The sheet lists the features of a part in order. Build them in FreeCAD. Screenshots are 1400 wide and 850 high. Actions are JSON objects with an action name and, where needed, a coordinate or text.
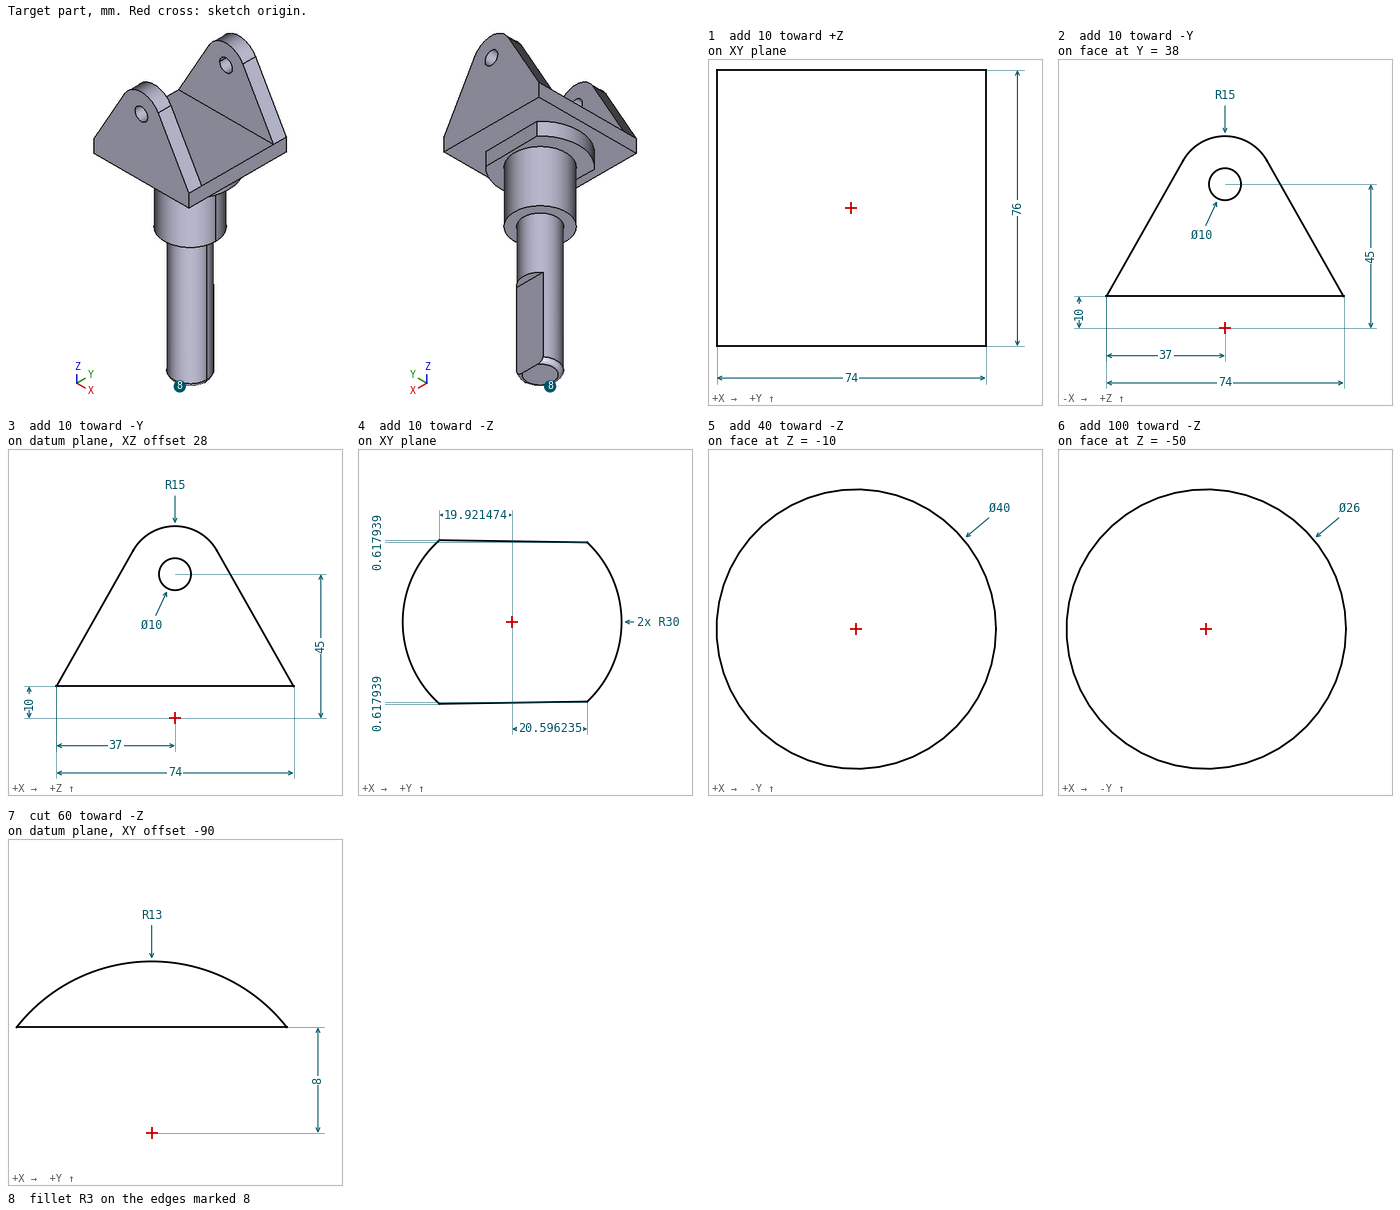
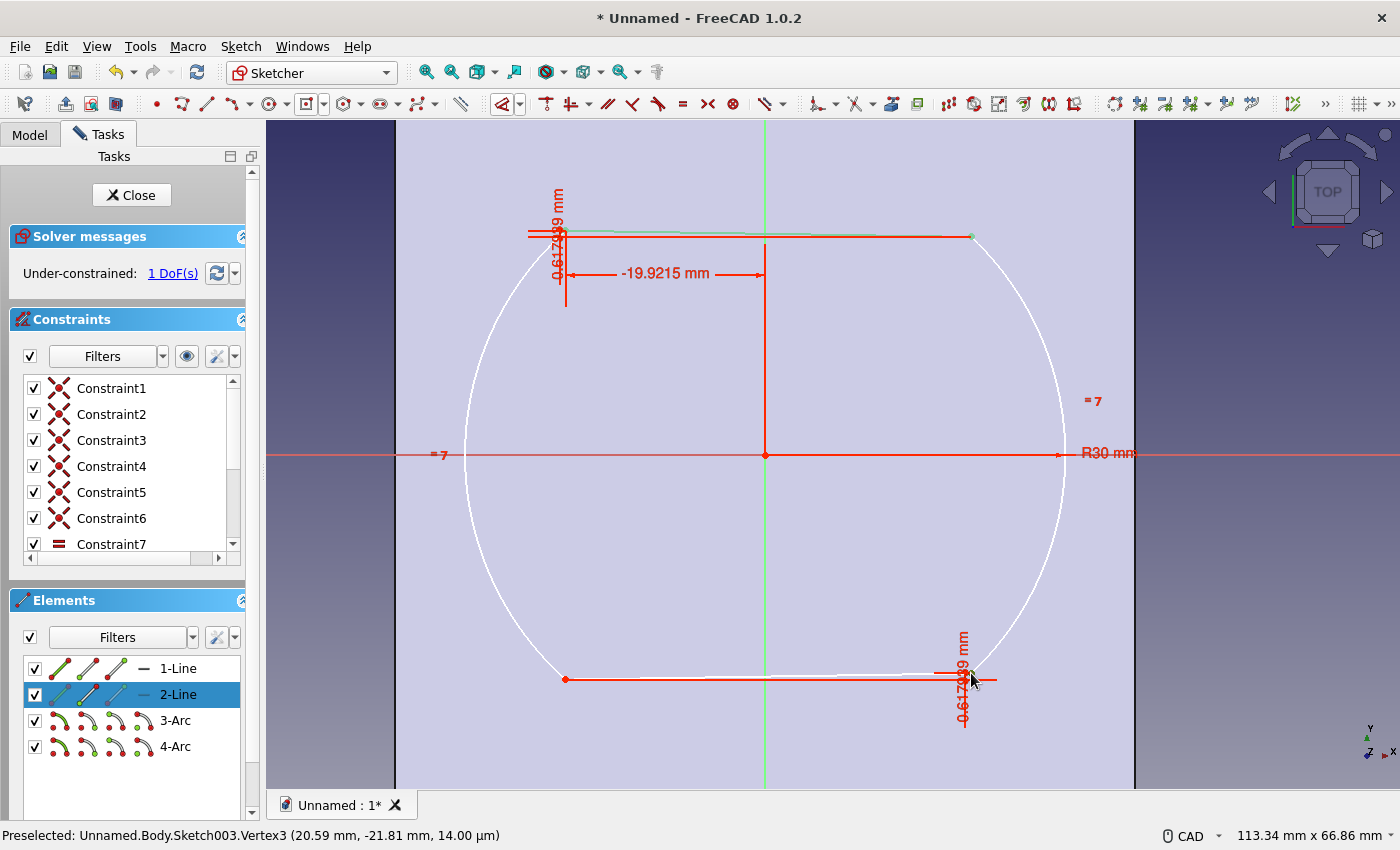
{"action": "left_click", "coordinate": [520, 104]}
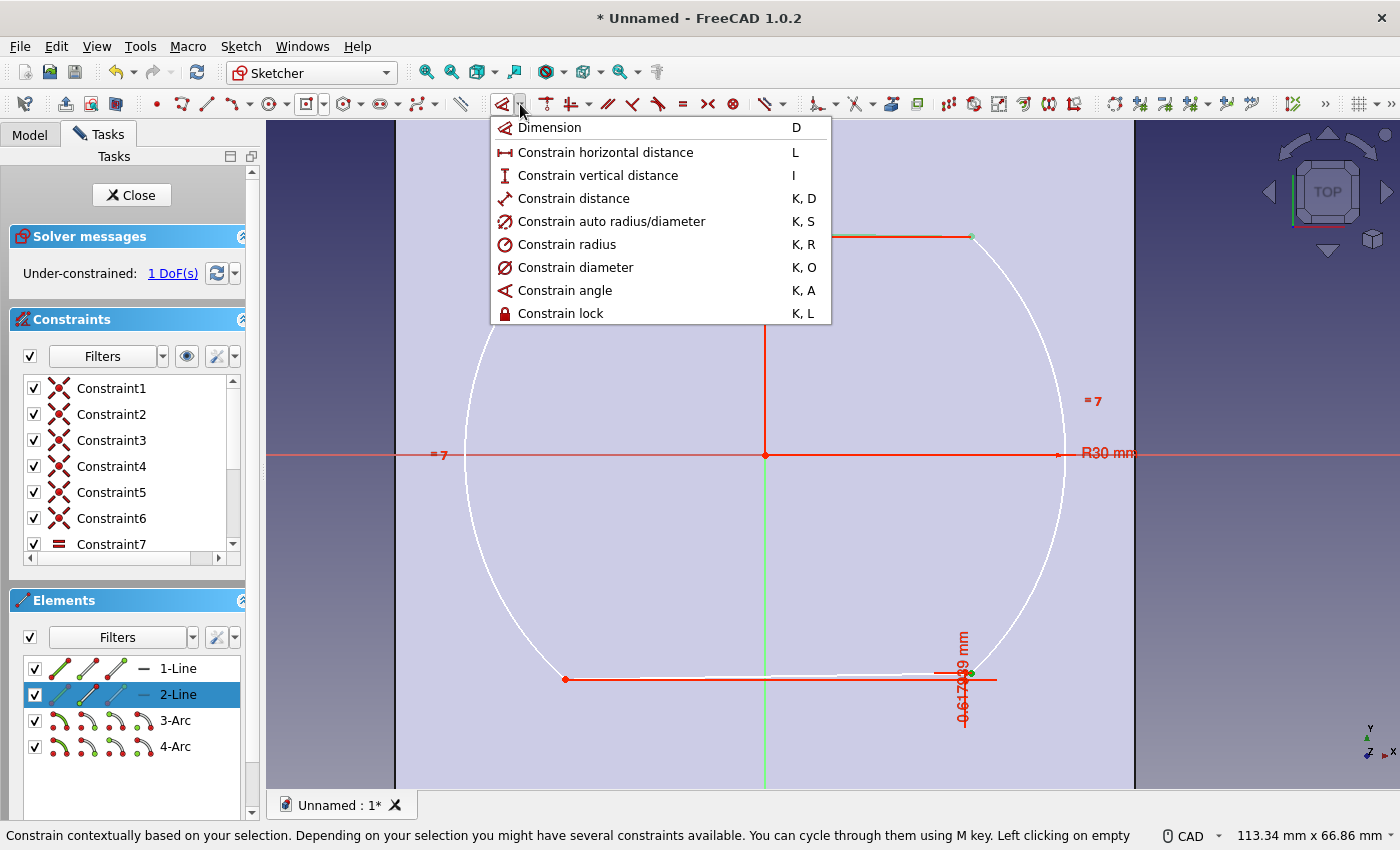
{"action": "left_click", "coordinate": [661, 152]}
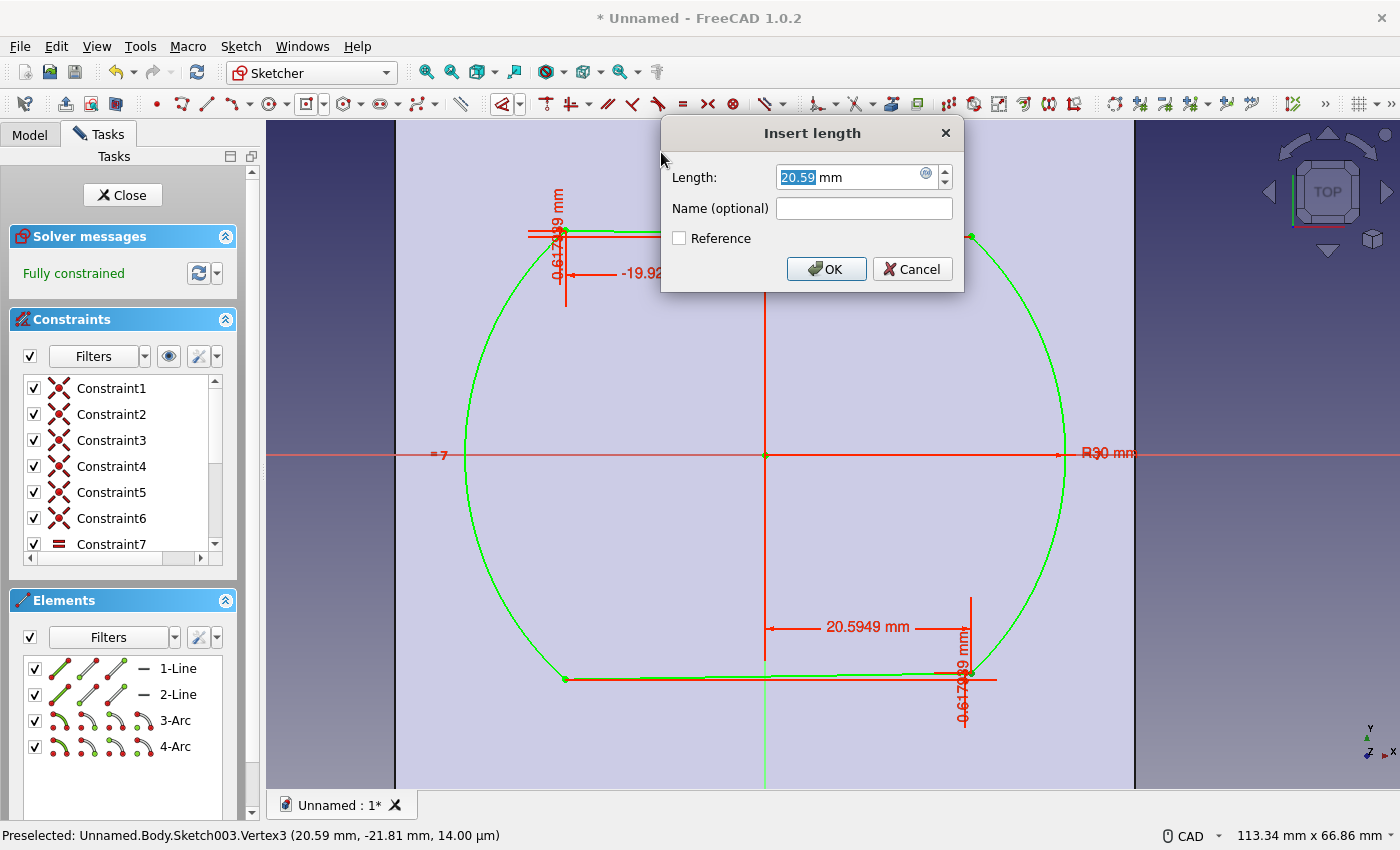
{"action": "type", "text": "20.596235"}
{"action": "key", "text": "Return"}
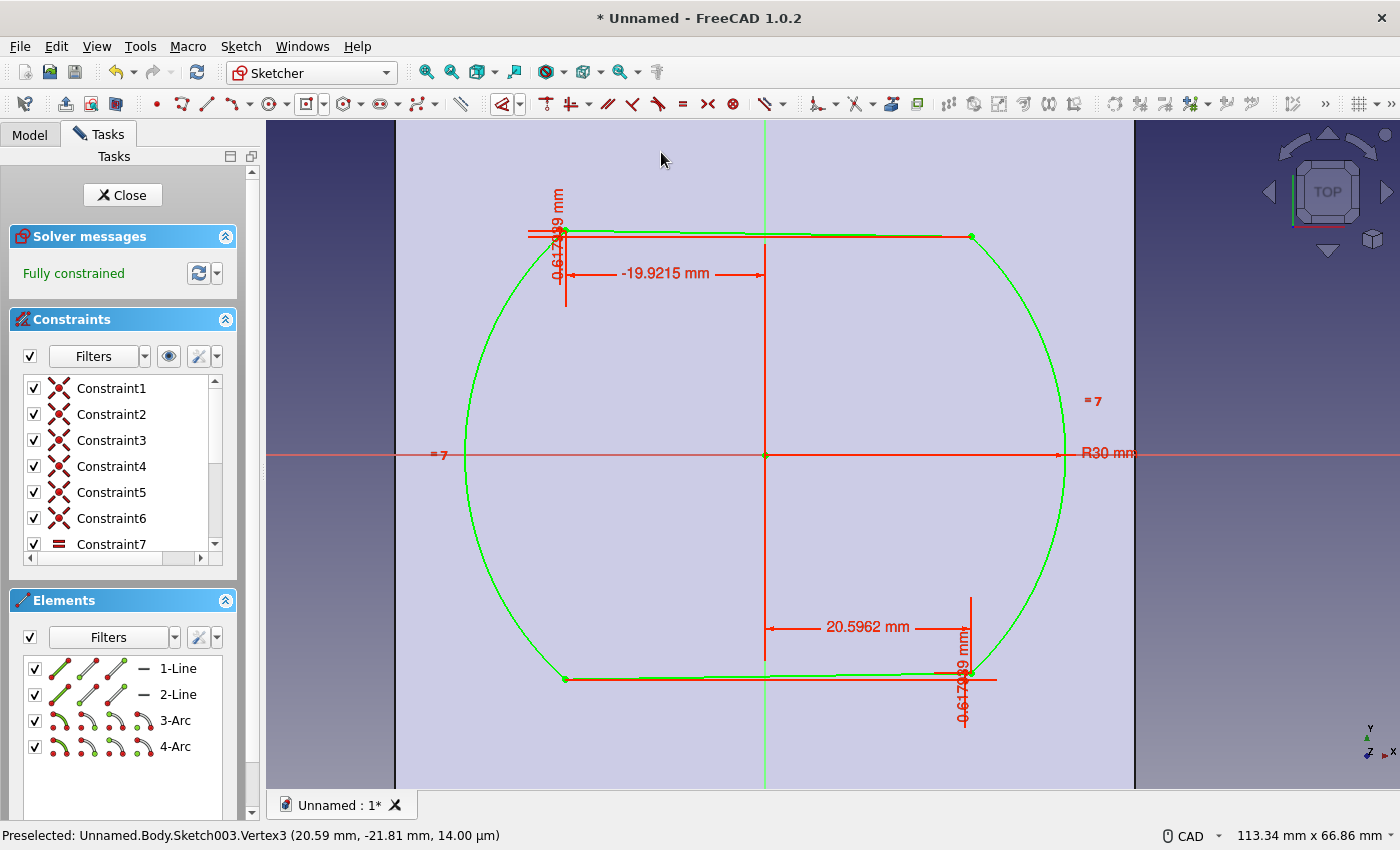
{"action": "left_click", "coordinate": [123, 195]}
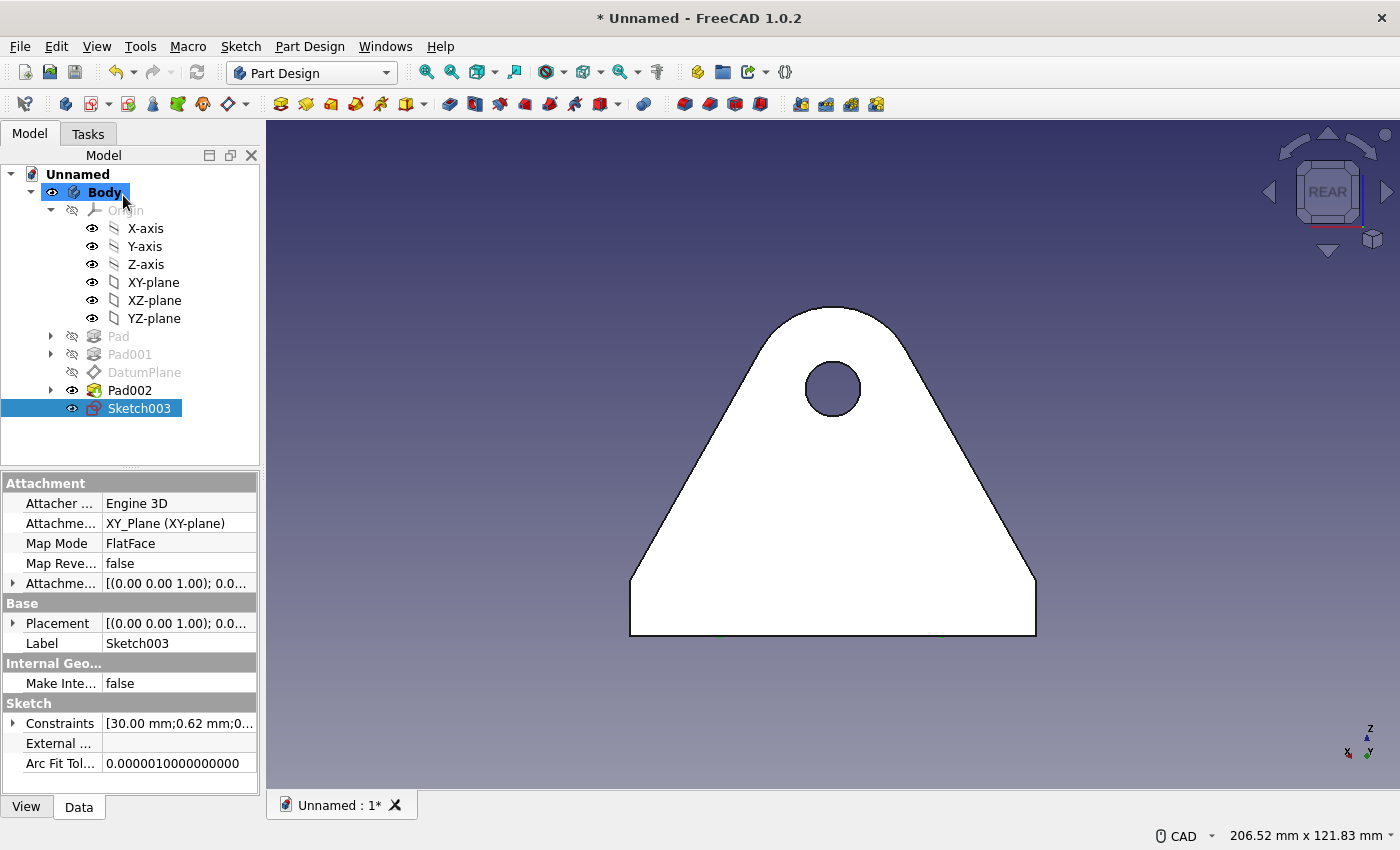
{"action": "left_click", "coordinate": [281, 104]}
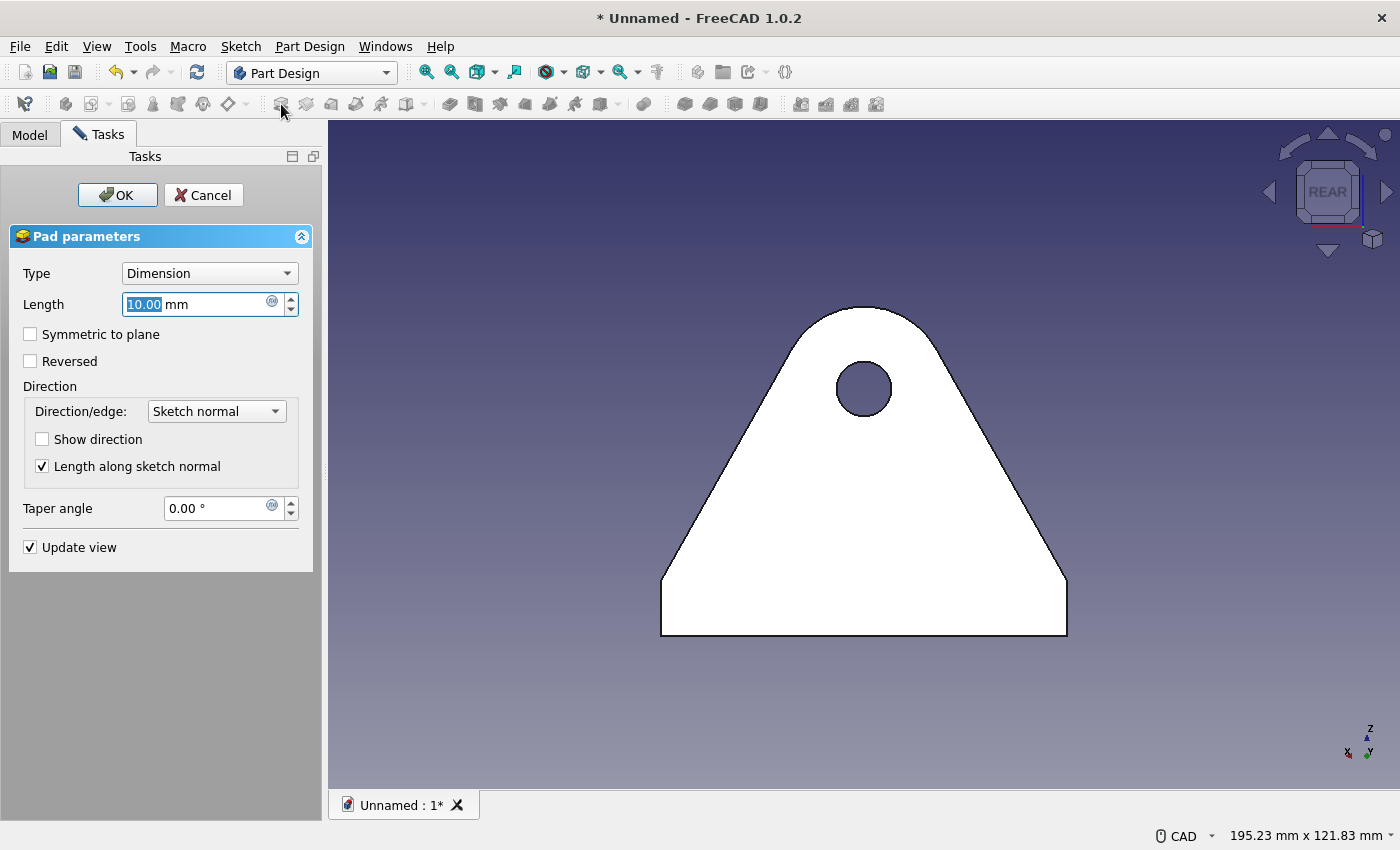
{"action": "type", "text": "10"}
{"action": "key", "text": "Tab"}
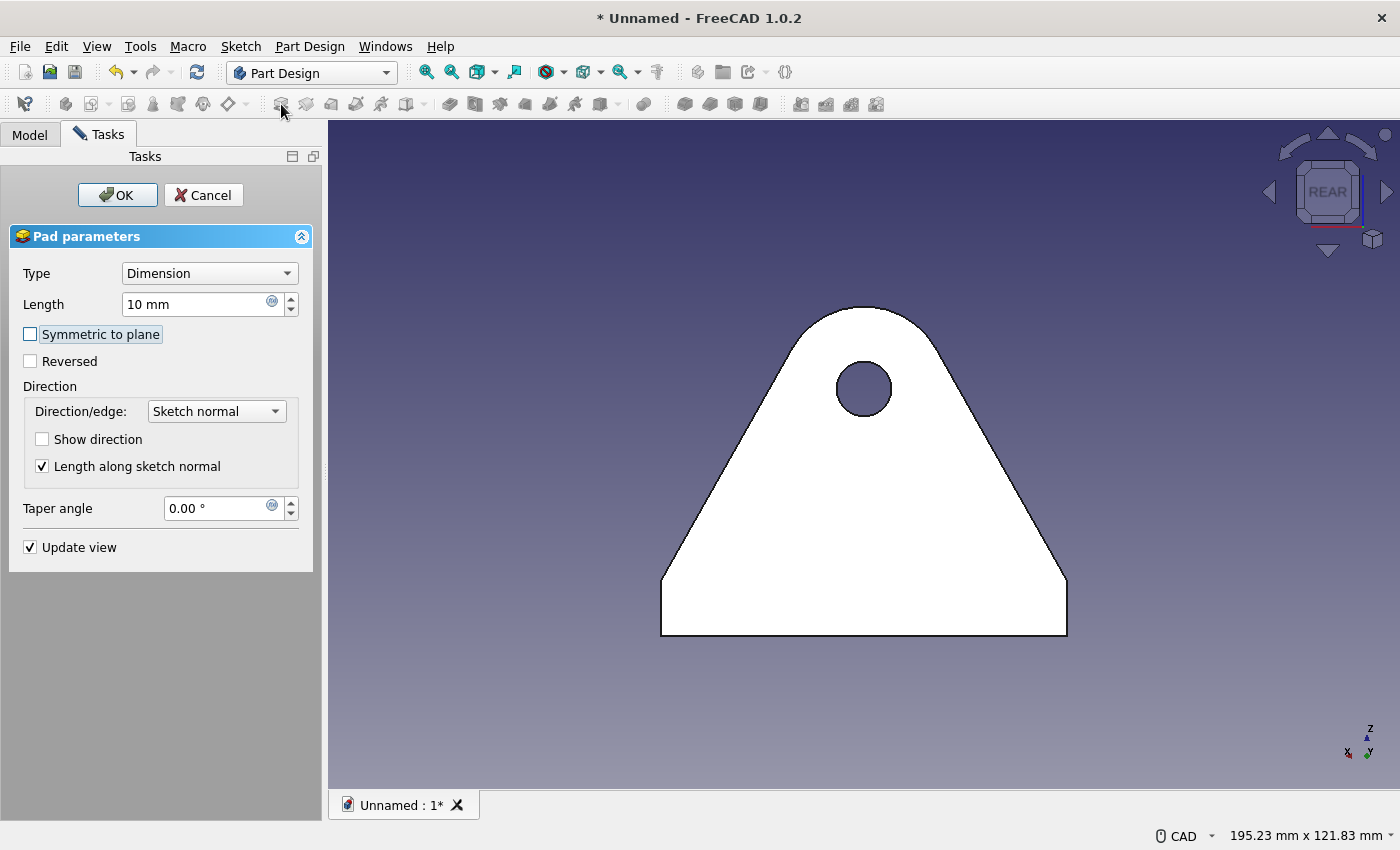
{"action": "left_click", "coordinate": [31, 361]}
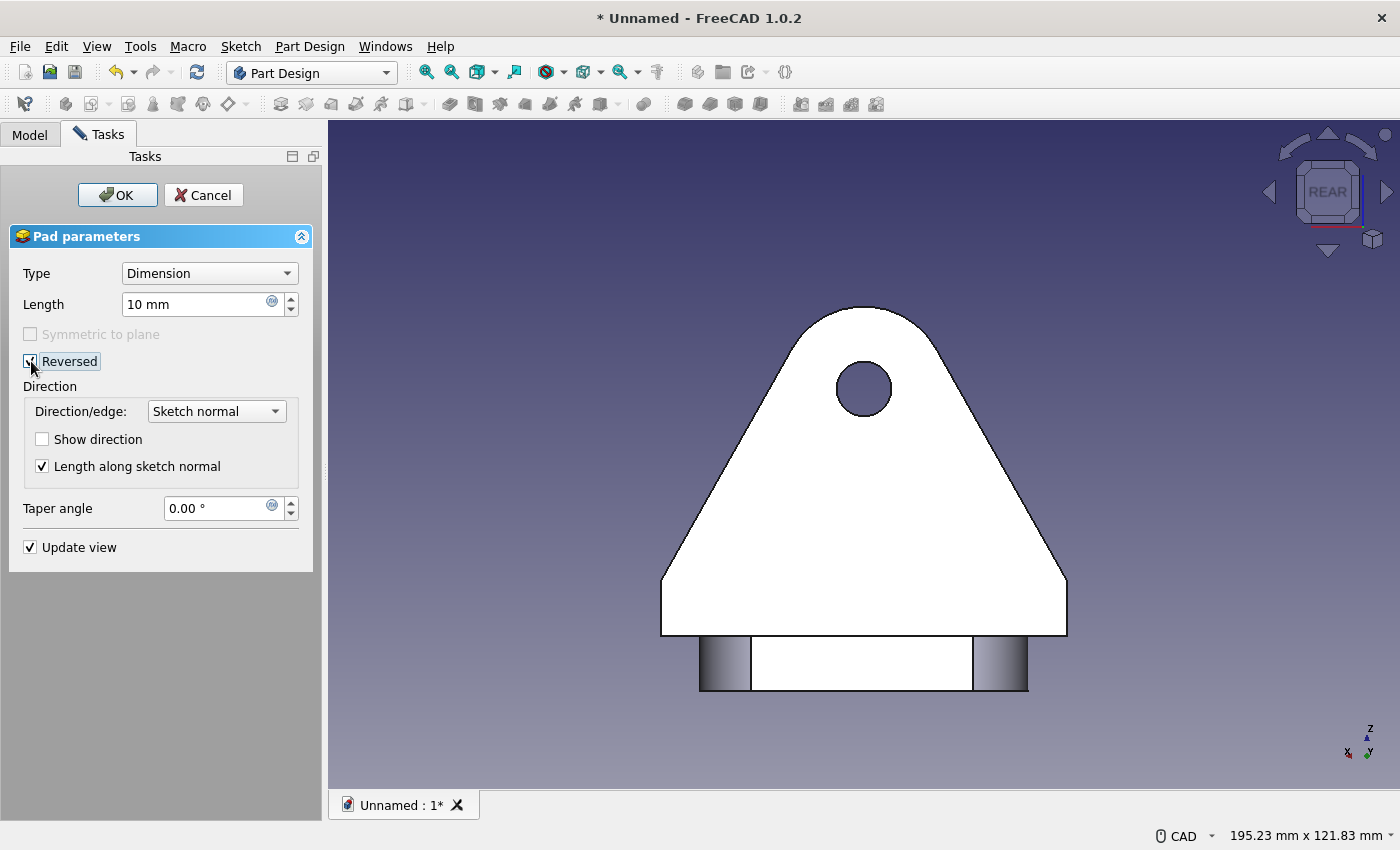
{"action": "left_click", "coordinate": [118, 195]}